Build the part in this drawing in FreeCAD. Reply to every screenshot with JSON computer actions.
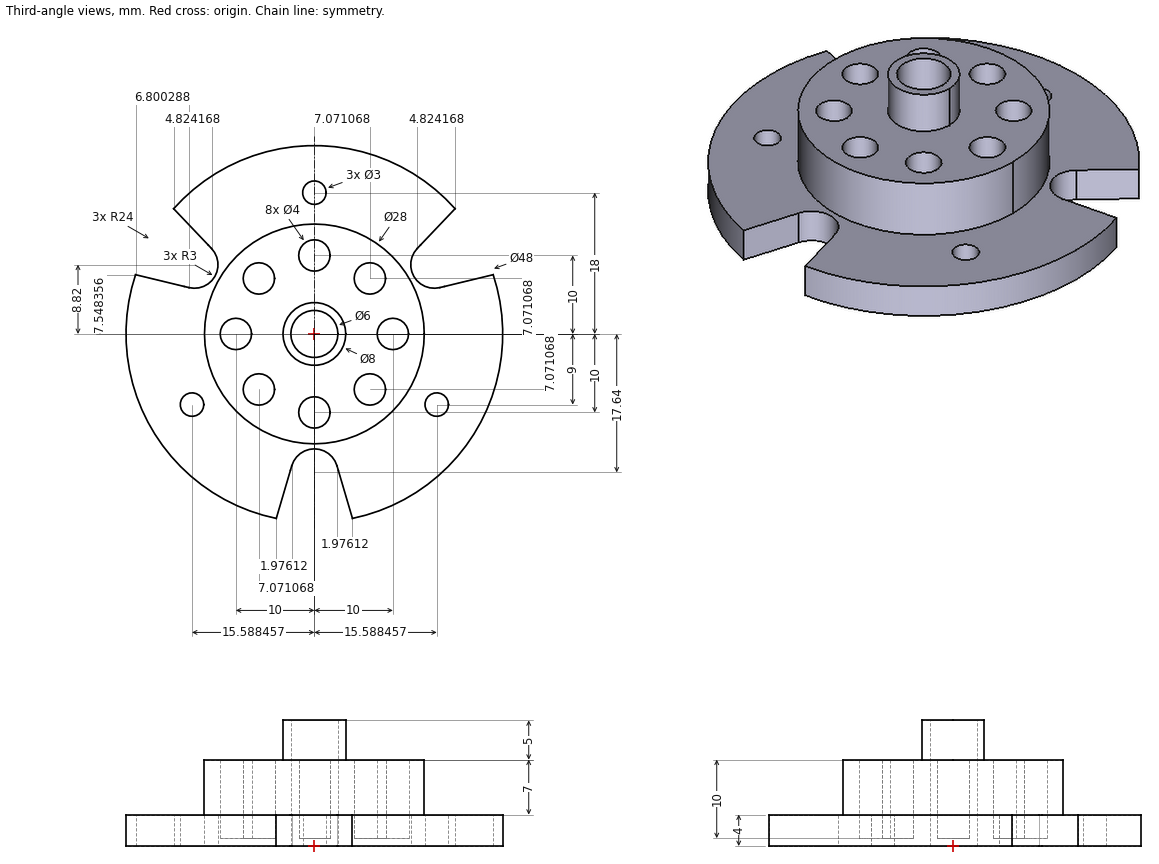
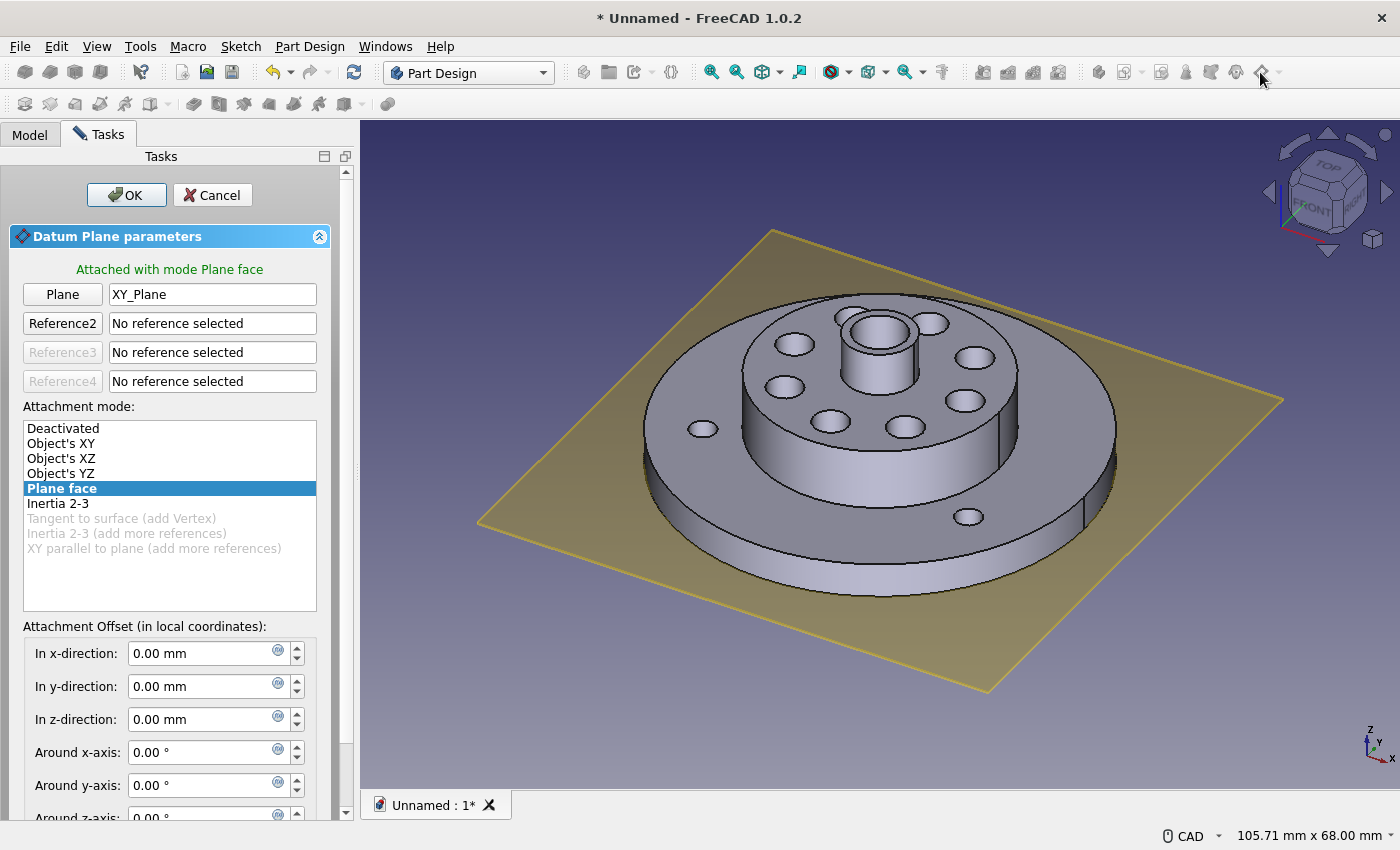
{"action": "triple_click", "coordinate": [210, 720]}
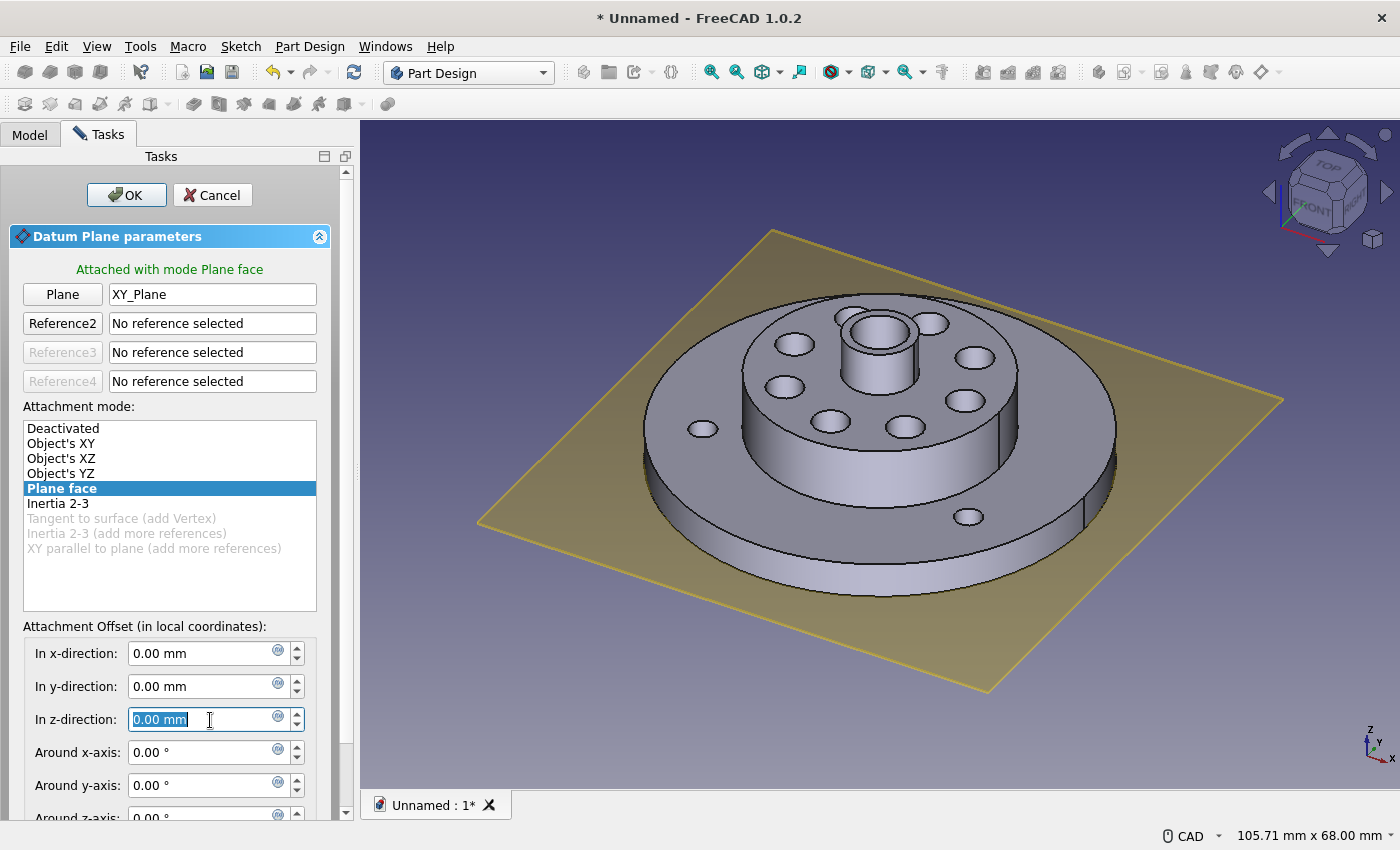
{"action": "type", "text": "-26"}
{"action": "key", "text": "Tab"}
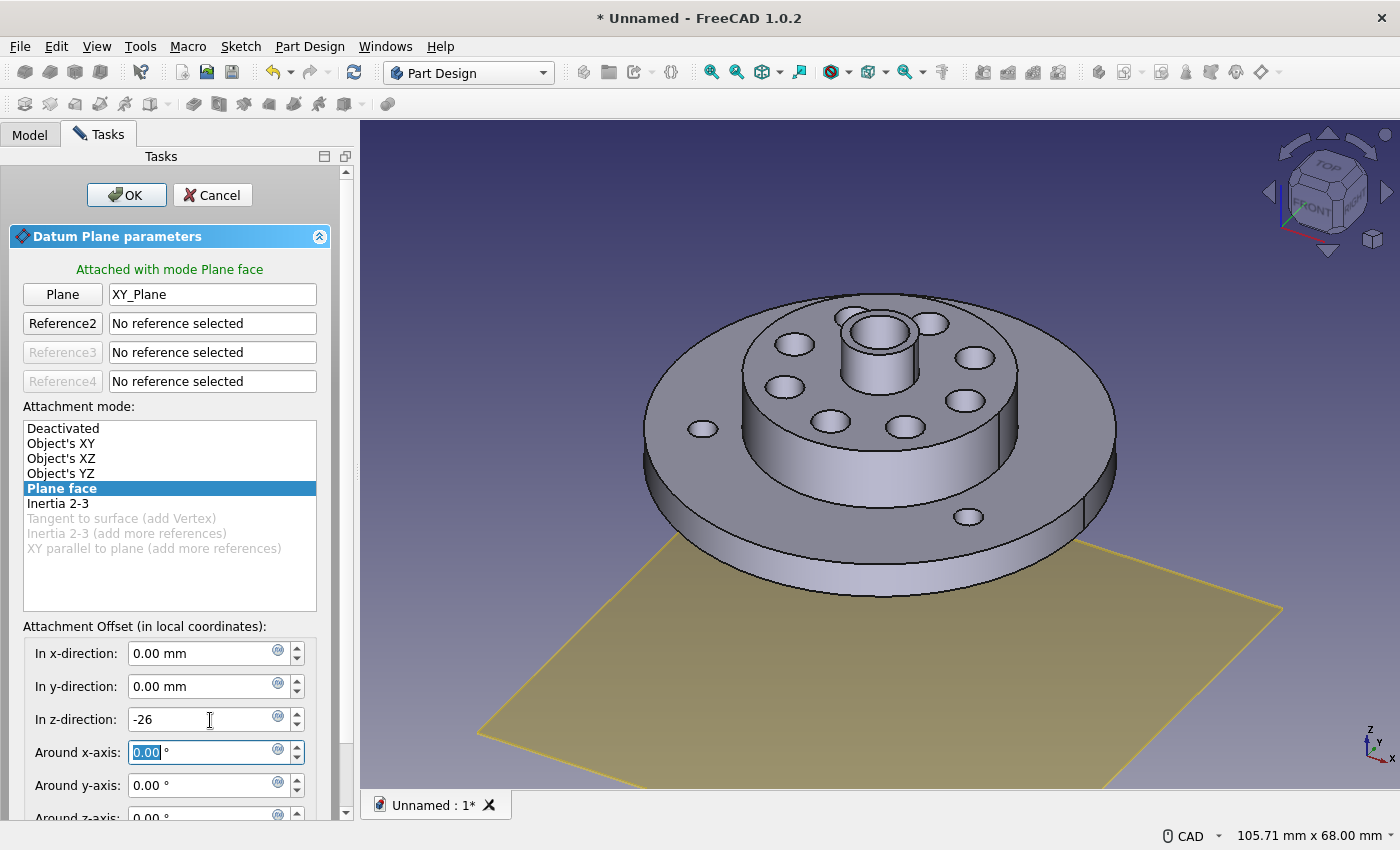
{"action": "left_click", "coordinate": [127, 195]}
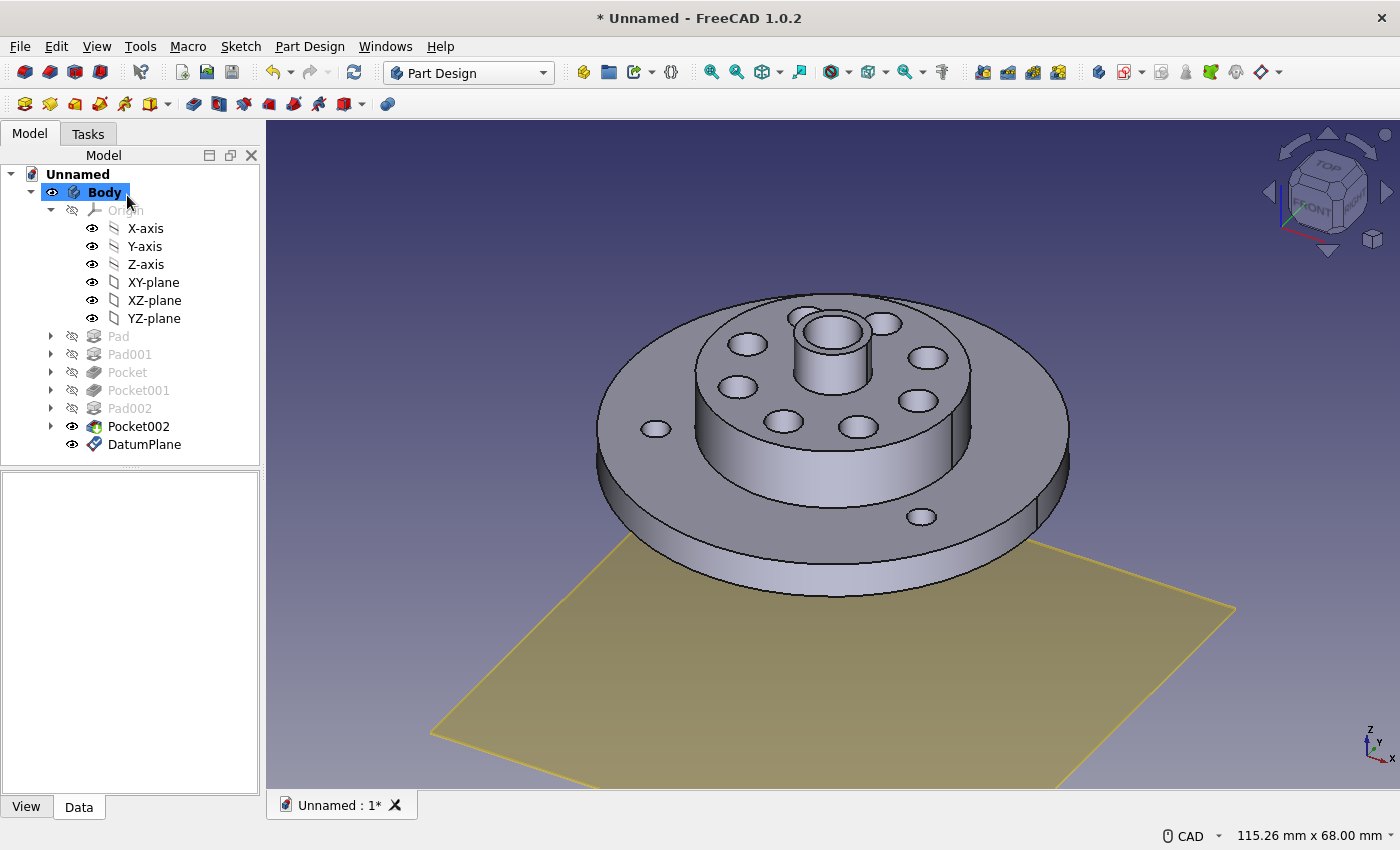
{"action": "left_click", "coordinate": [117, 444]}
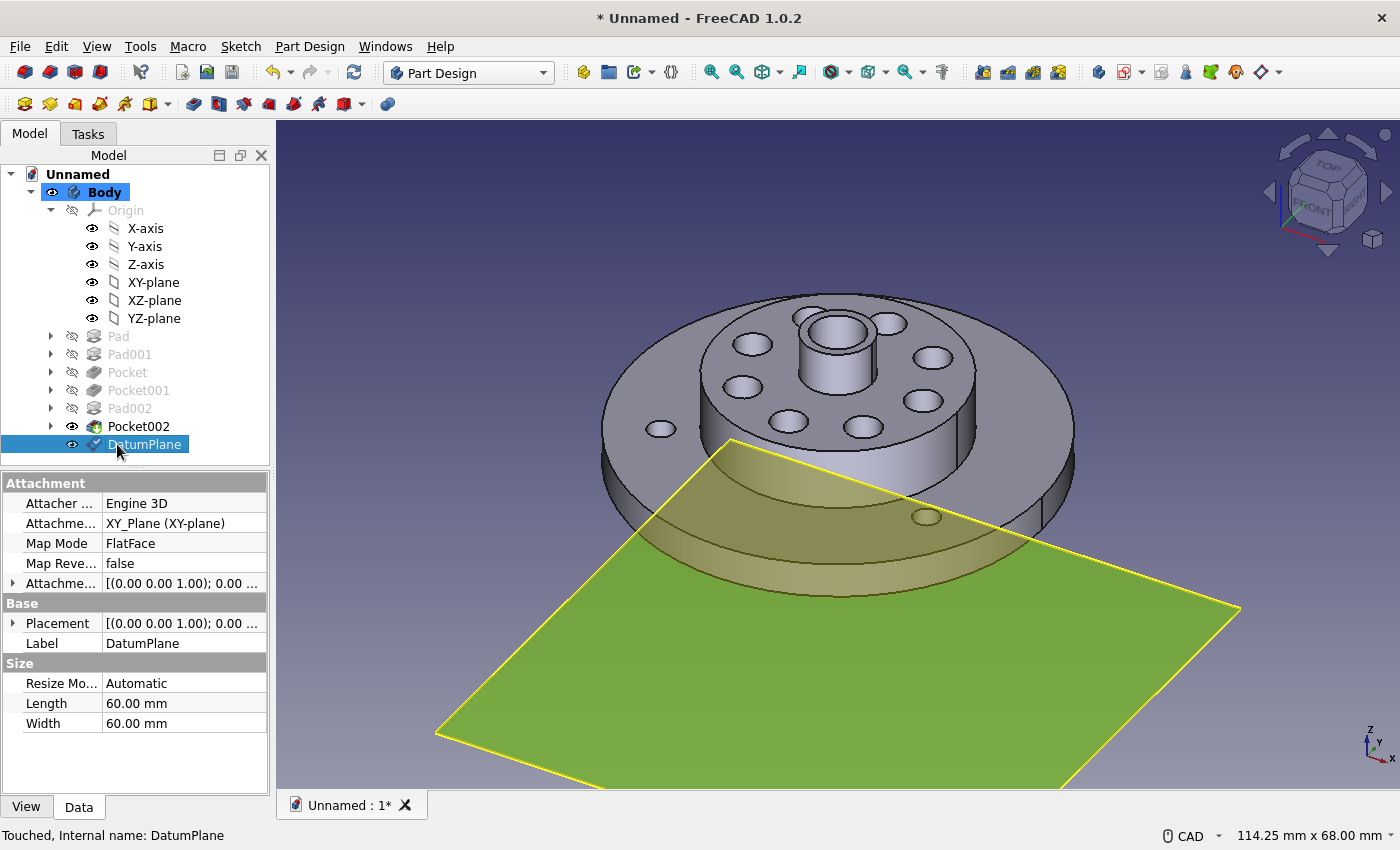
{"action": "left_click", "coordinate": [1124, 72]}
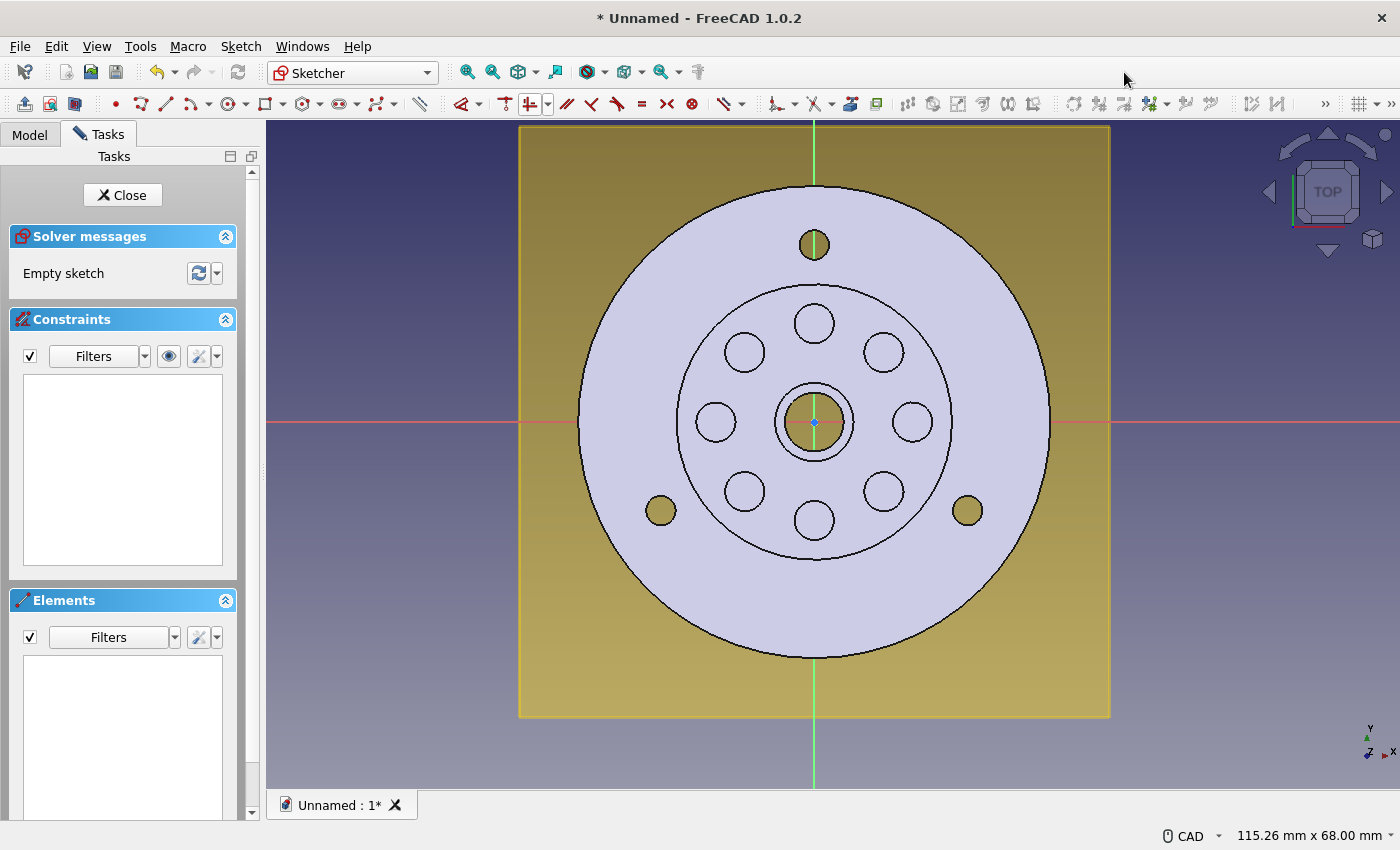
{"action": "key", "text": "q s"}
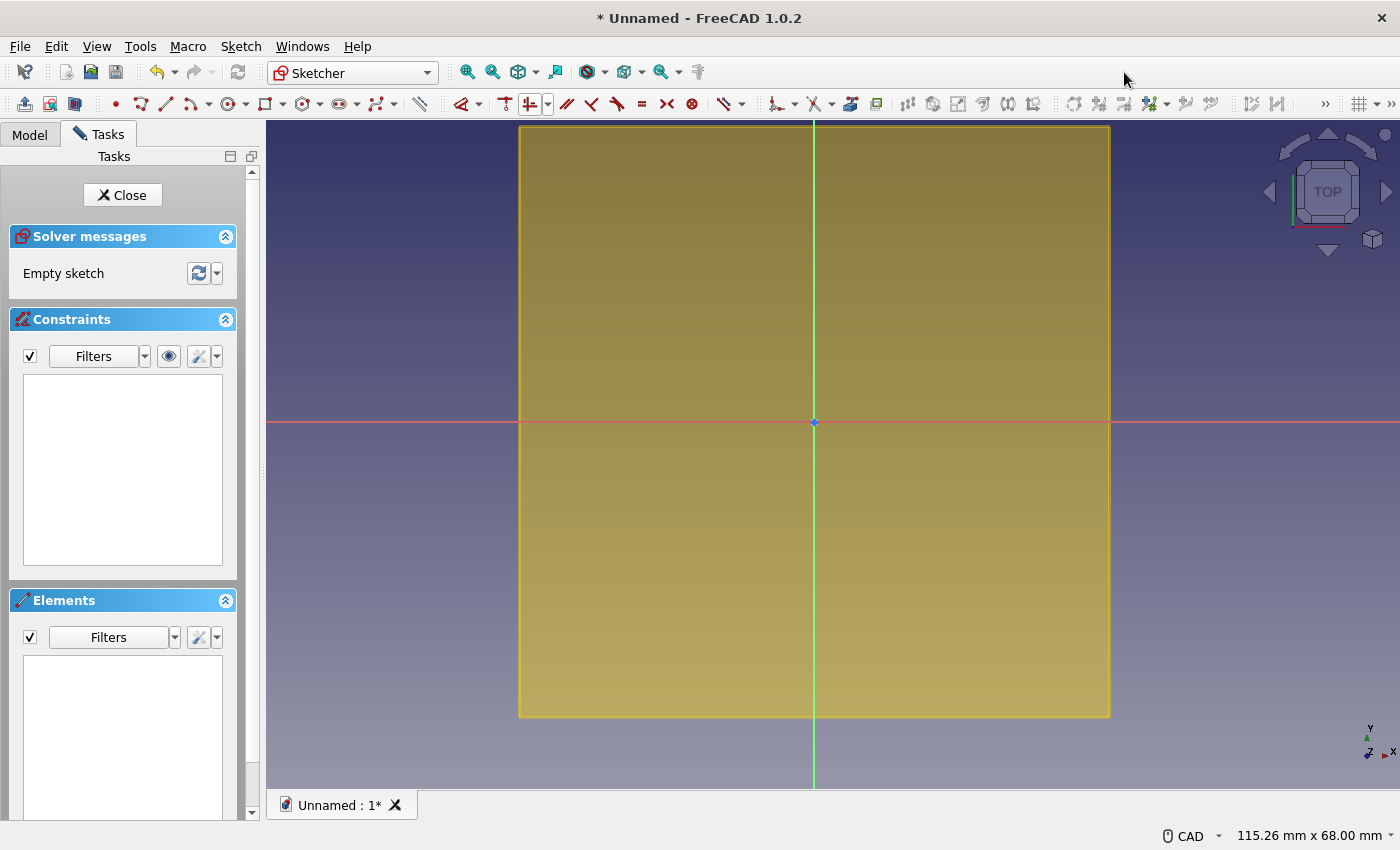
{"action": "left_click", "coordinate": [166, 104]}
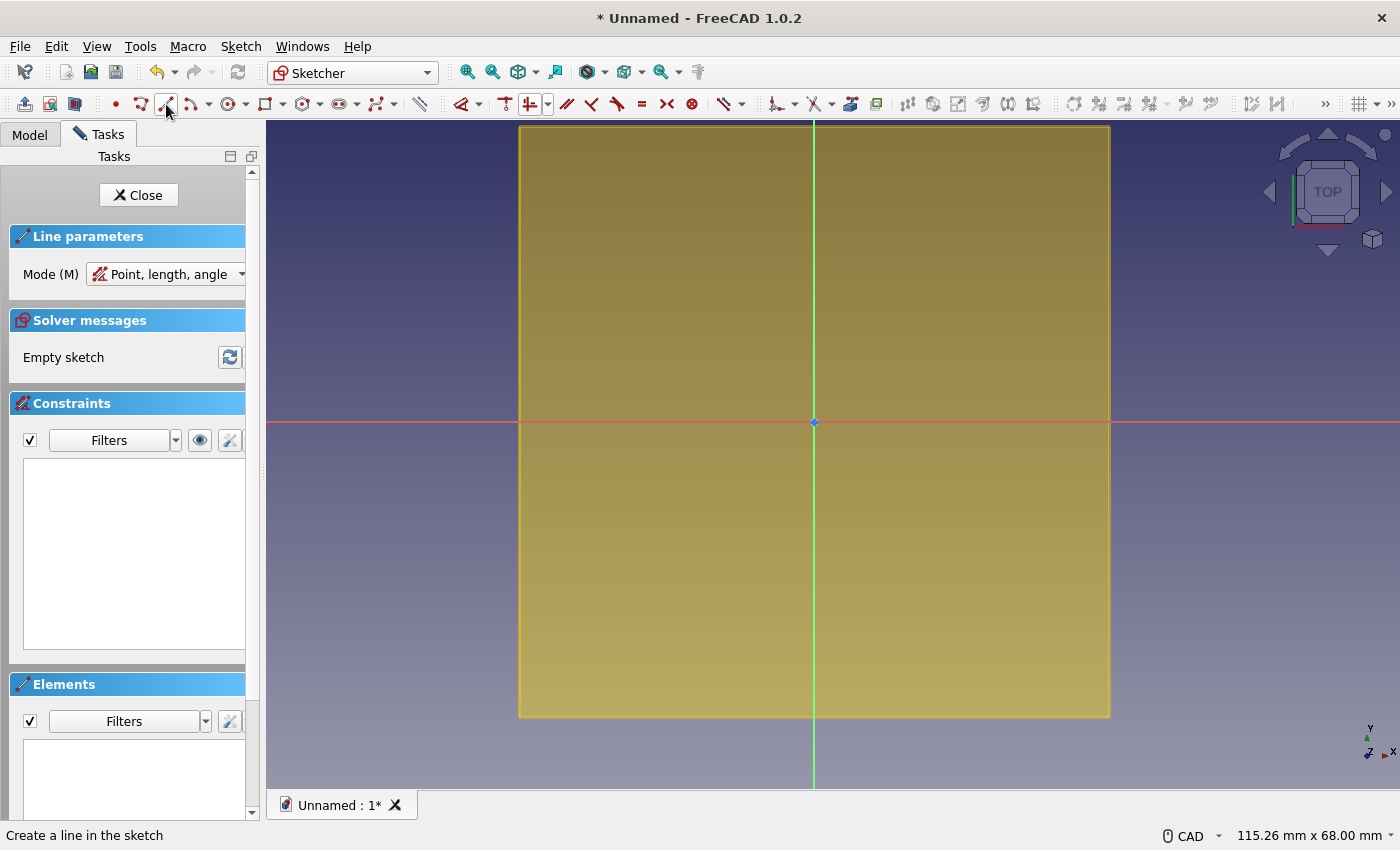
{"action": "left_click", "coordinate": [590, 348]}
{"action": "left_click", "coordinate": [657, 364]}